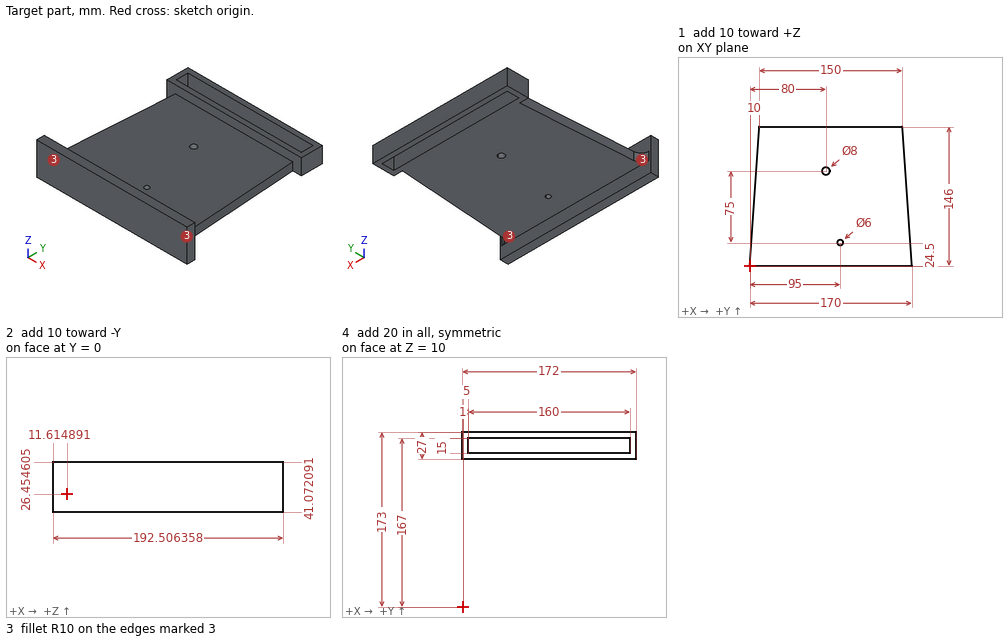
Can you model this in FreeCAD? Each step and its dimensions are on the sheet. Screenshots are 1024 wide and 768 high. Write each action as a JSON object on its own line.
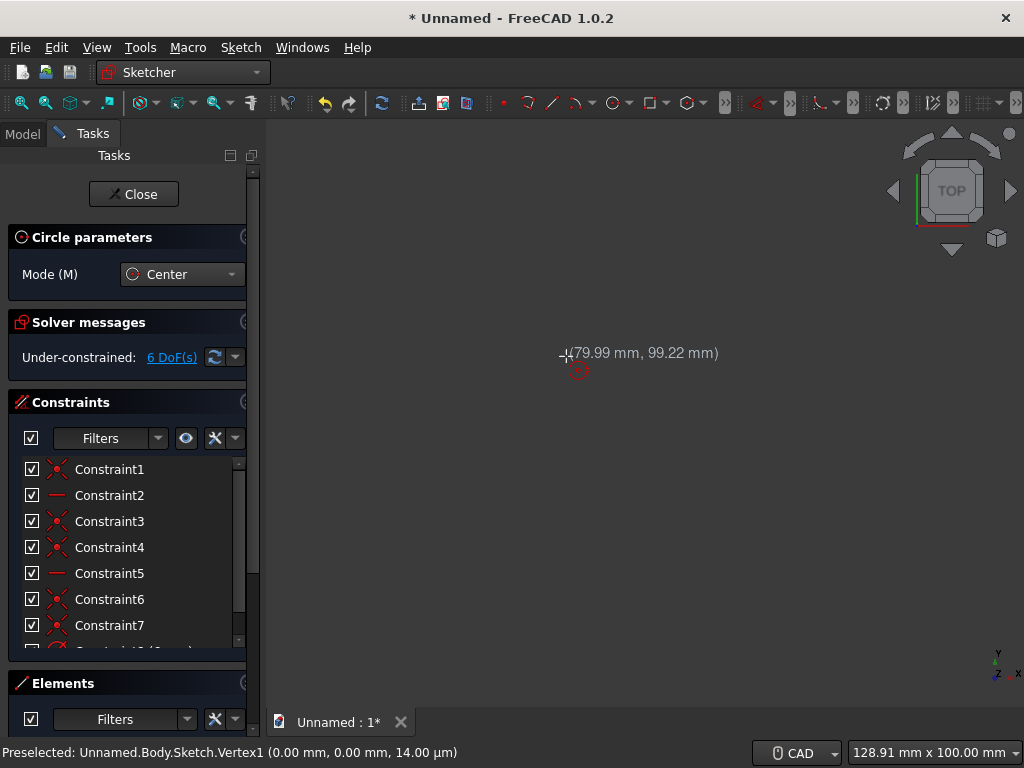
{"action": "left_click", "coordinate": [565, 356]}
{"action": "mouse_move", "coordinate": [582, 340]}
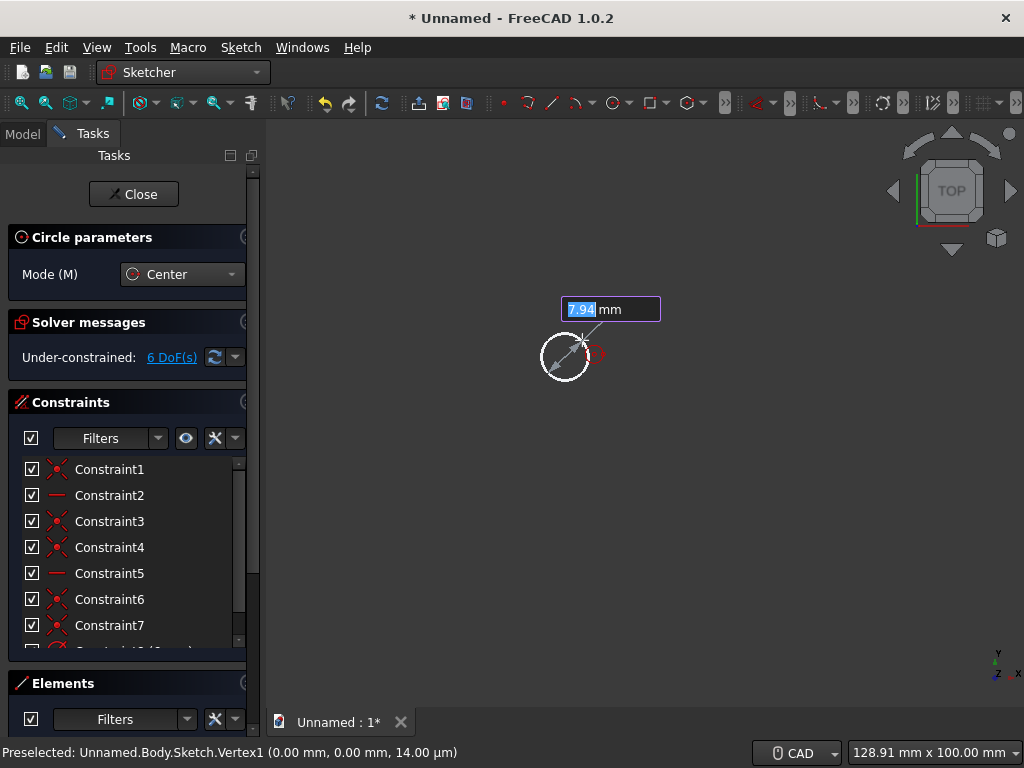
{"action": "type", "text": "8"}
{"action": "key", "text": "Return"}
{"action": "key", "text": "Escape"}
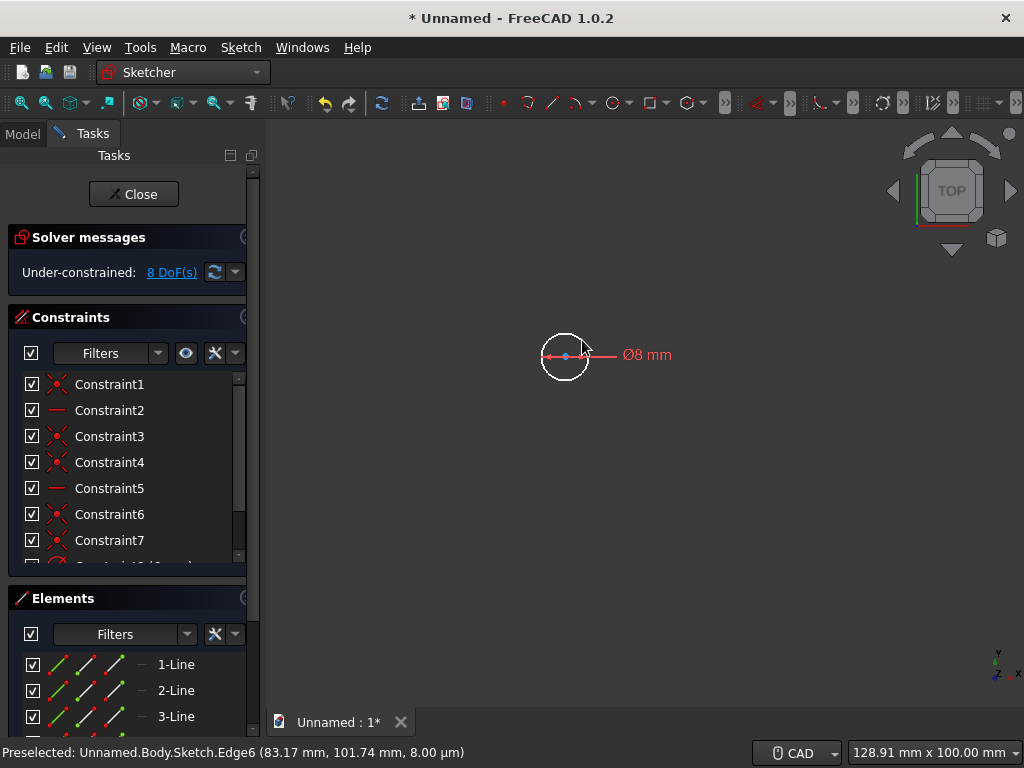
{"action": "left_click", "coordinate": [756, 104]}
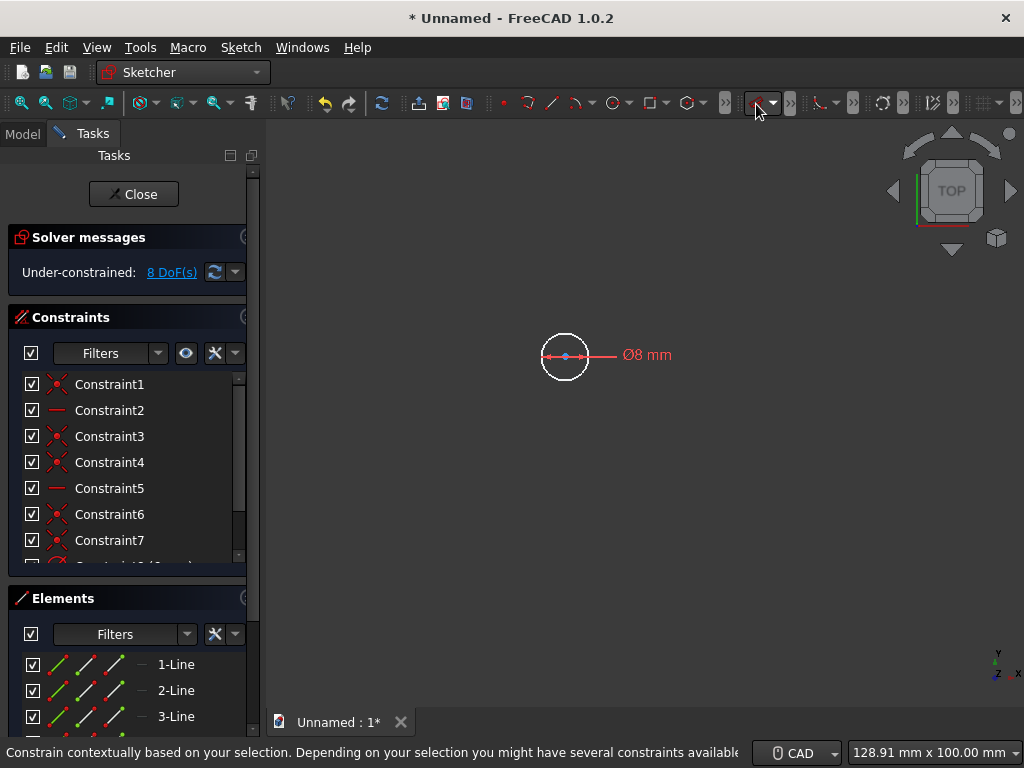
{"action": "scroll", "coordinate": [566, 355], "scroll_direction": "down", "scroll_amount": 5}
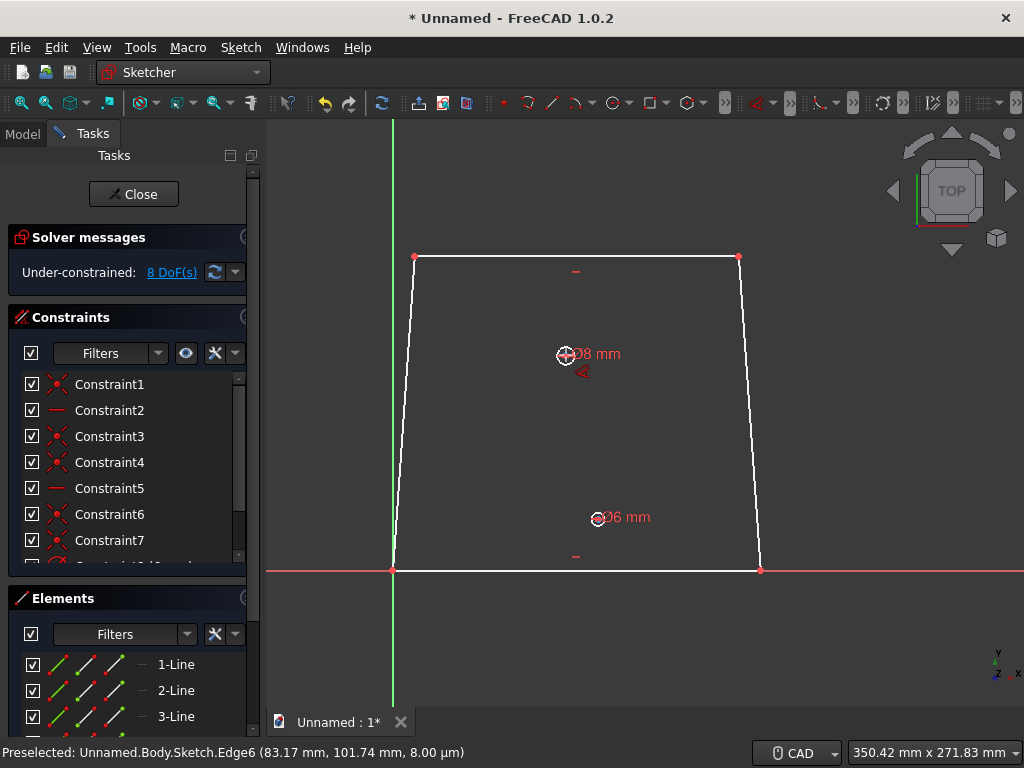
{"action": "left_click", "coordinate": [598, 519]}
{"action": "left_click", "coordinate": [495, 605]}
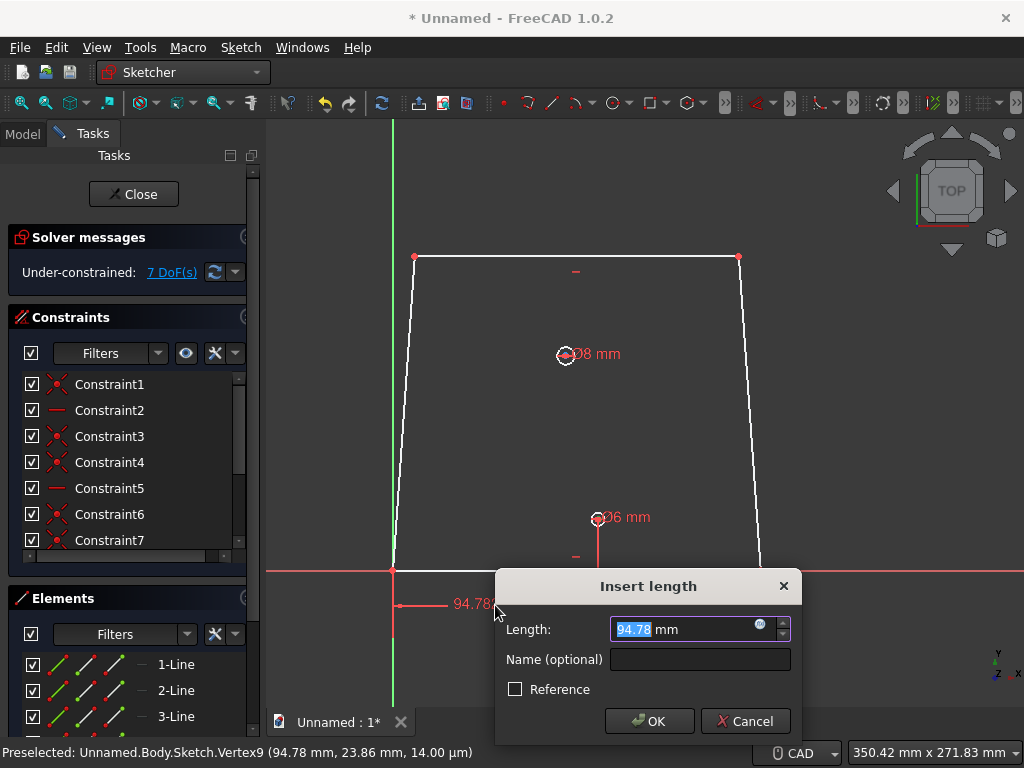
{"action": "type", "text": "95"}
{"action": "key", "text": "Return"}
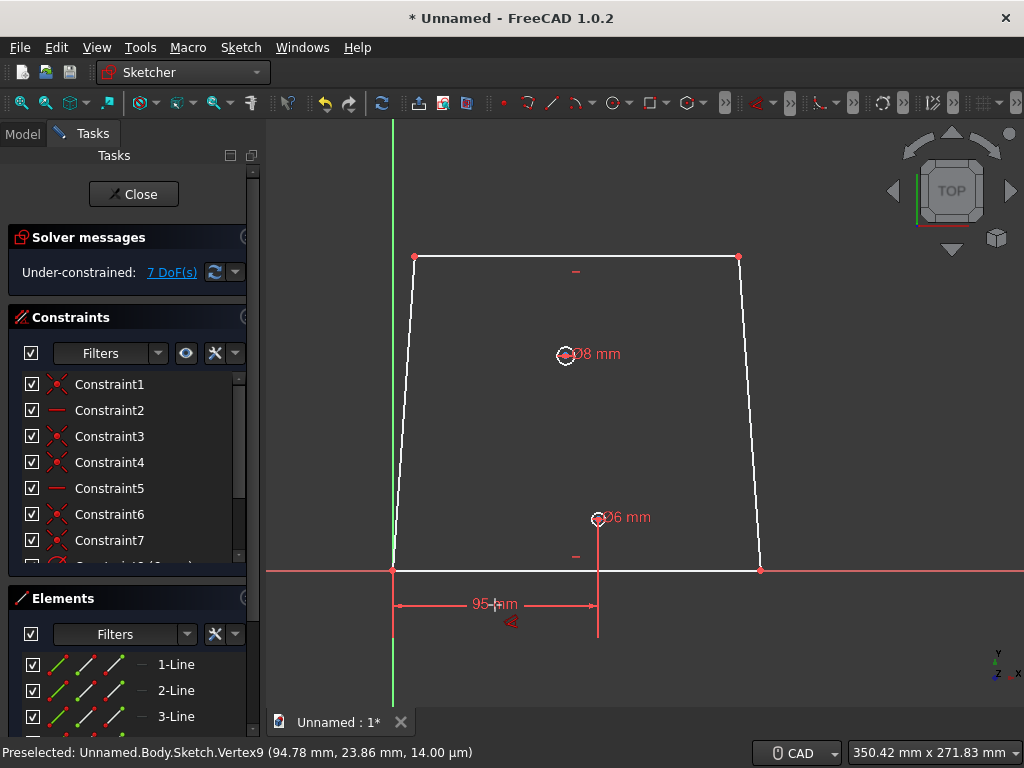
{"action": "left_click", "coordinate": [566, 356]}
{"action": "left_click", "coordinate": [419, 605]}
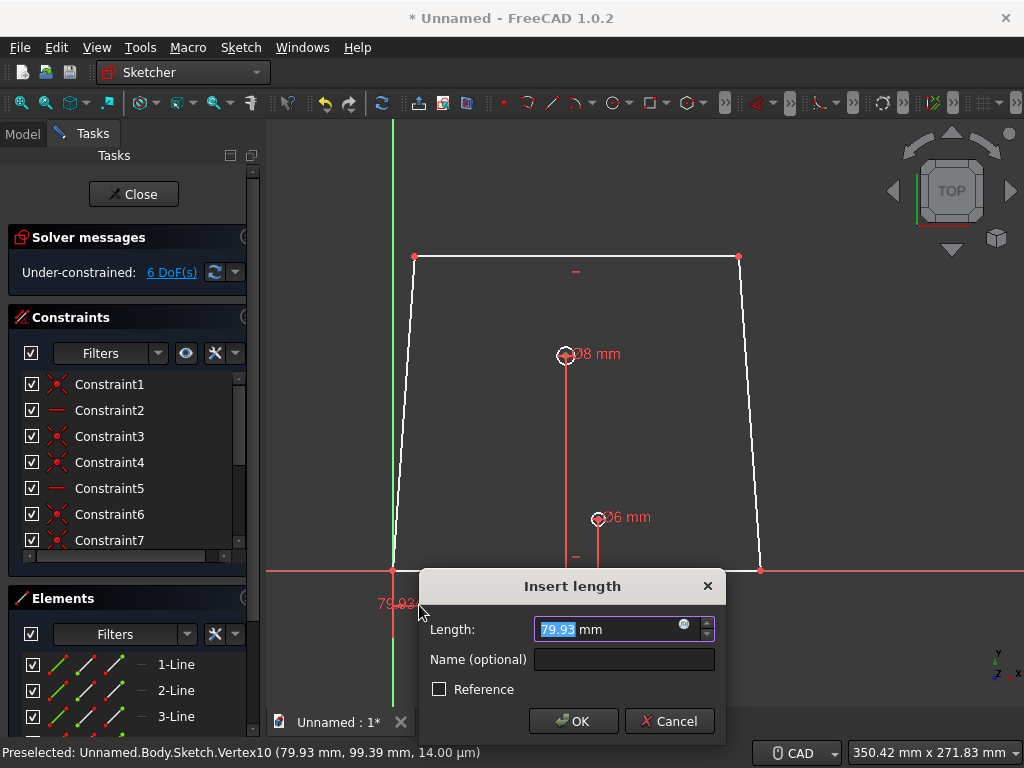
{"action": "type", "text": "80"}
{"action": "key", "text": "Return"}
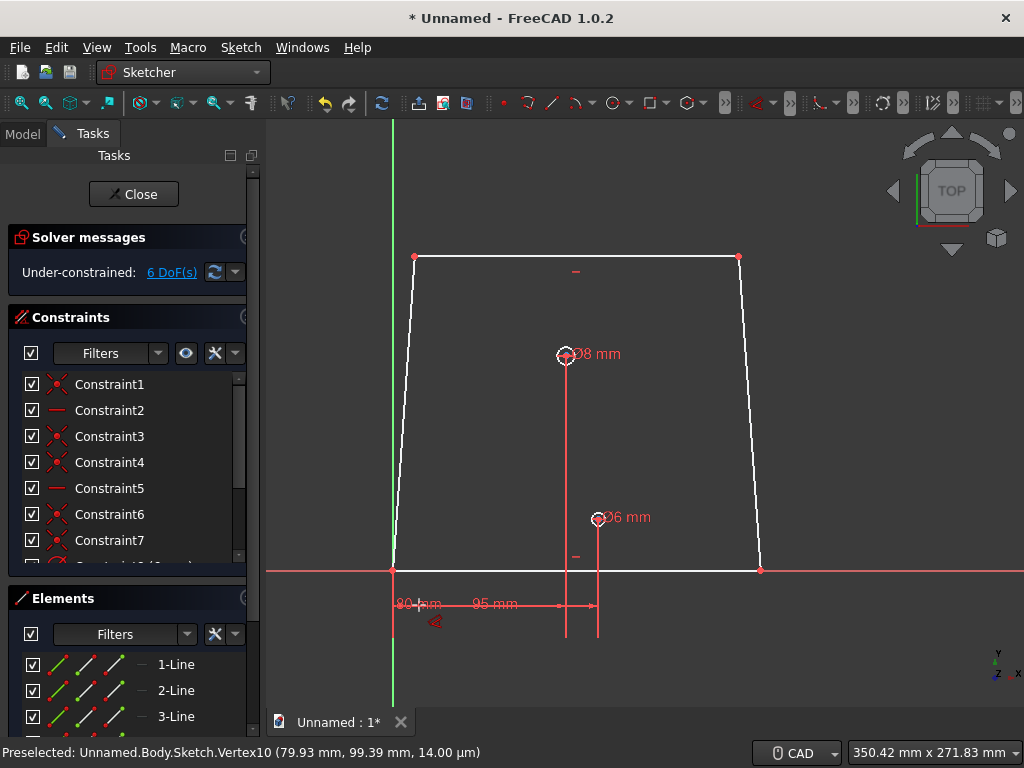
{"action": "left_click", "coordinate": [503, 571]}
{"action": "left_click", "coordinate": [577, 605]}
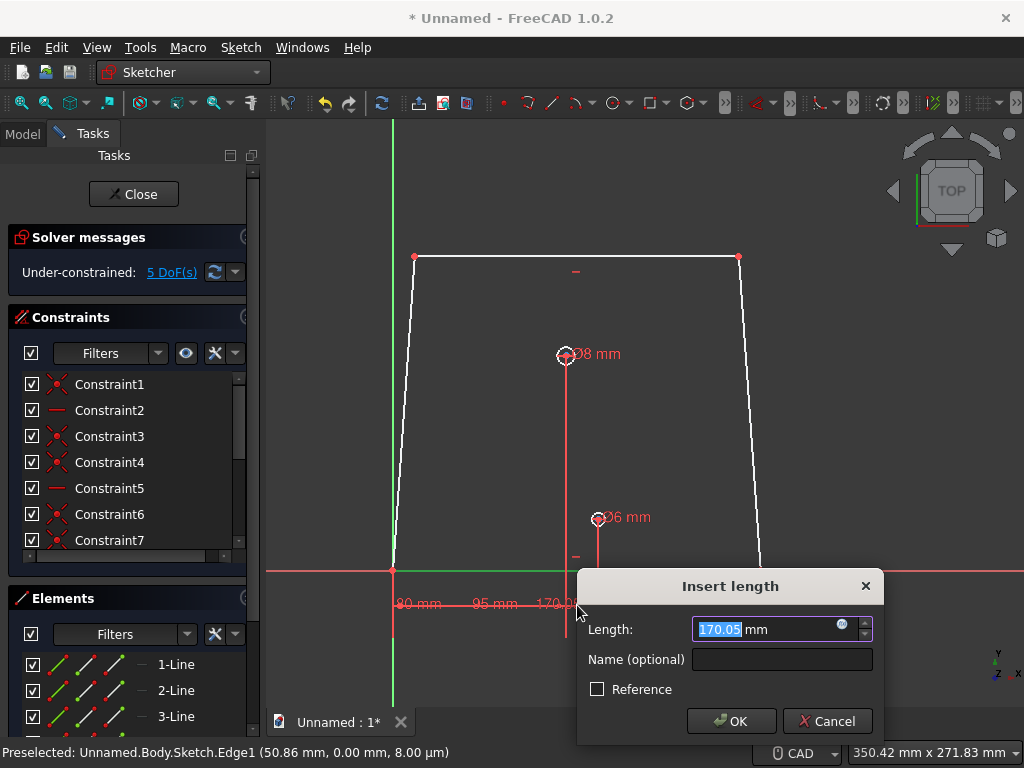
{"action": "type", "text": "170"}
{"action": "key", "text": "Return"}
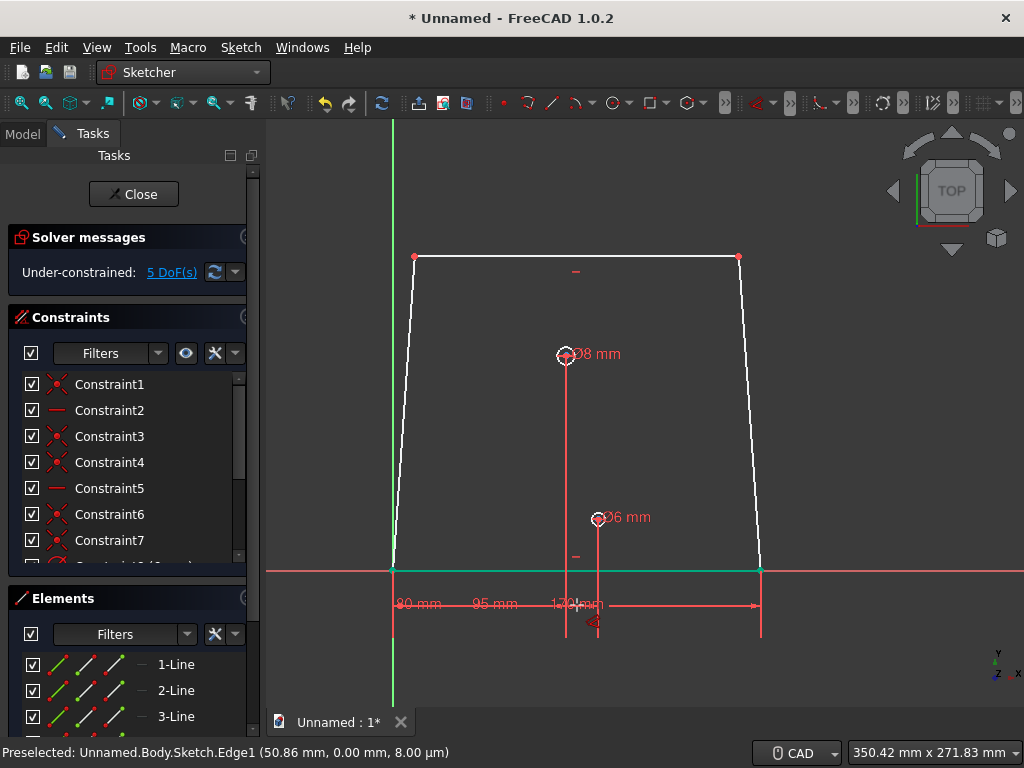
{"action": "left_click", "coordinate": [642, 256]}
{"action": "left_click", "coordinate": [577, 222]}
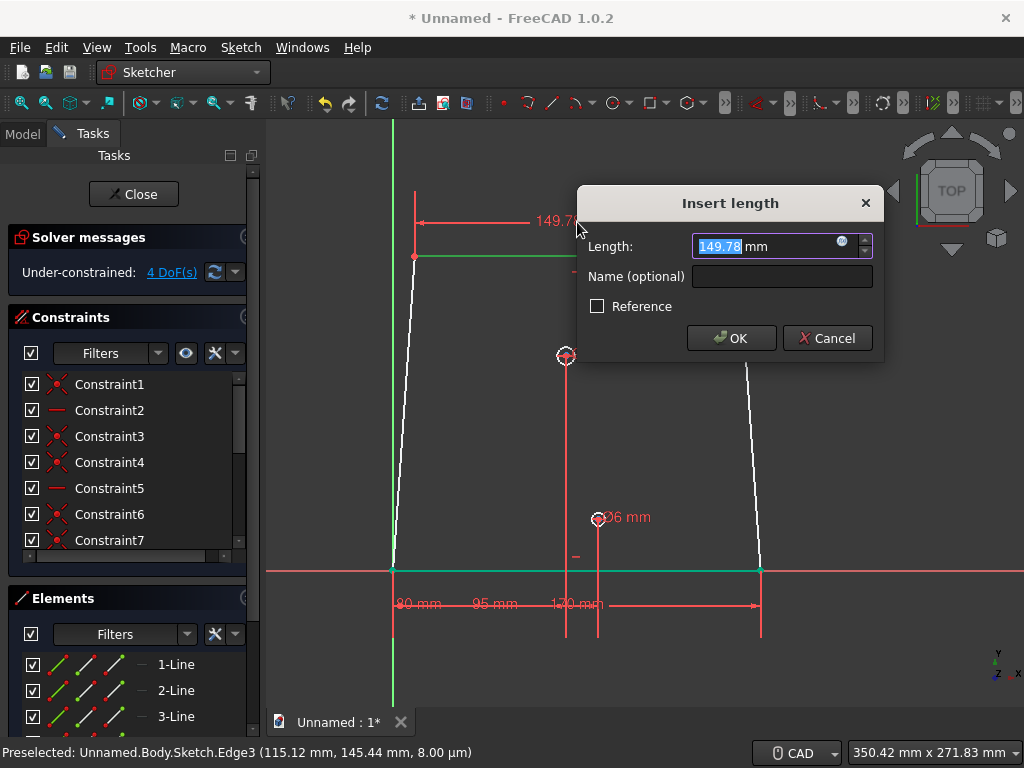
{"action": "type", "text": "150"}
{"action": "key", "text": "Return"}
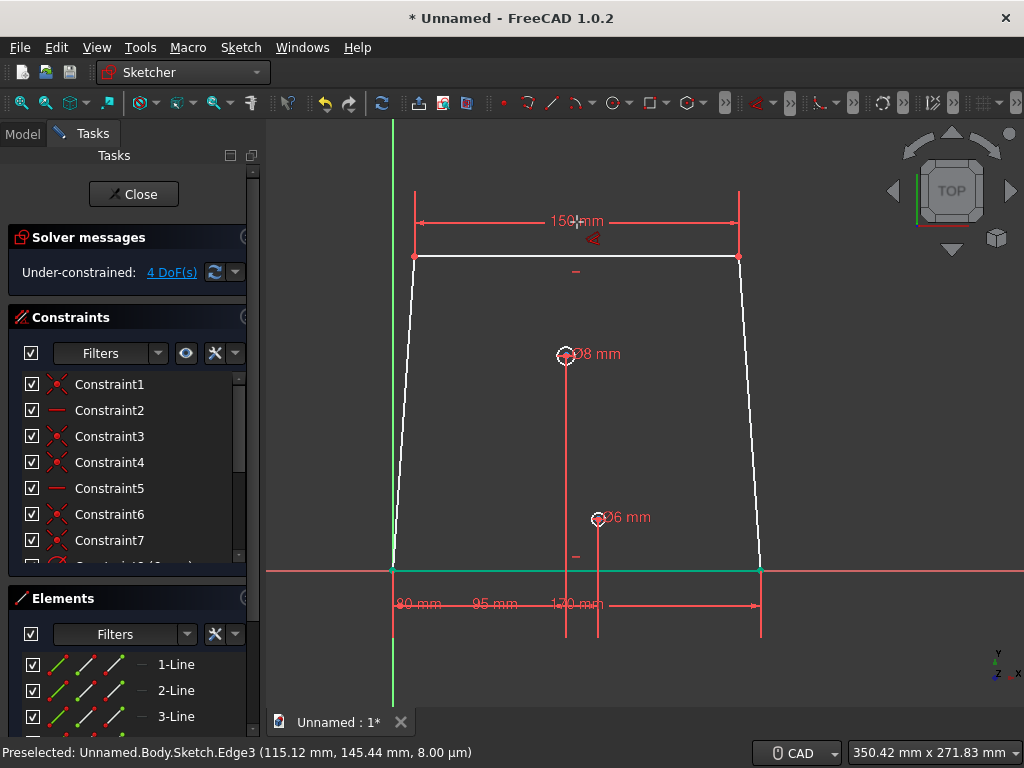
{"action": "scroll", "coordinate": [415, 256], "scroll_direction": "up", "scroll_amount": 4}